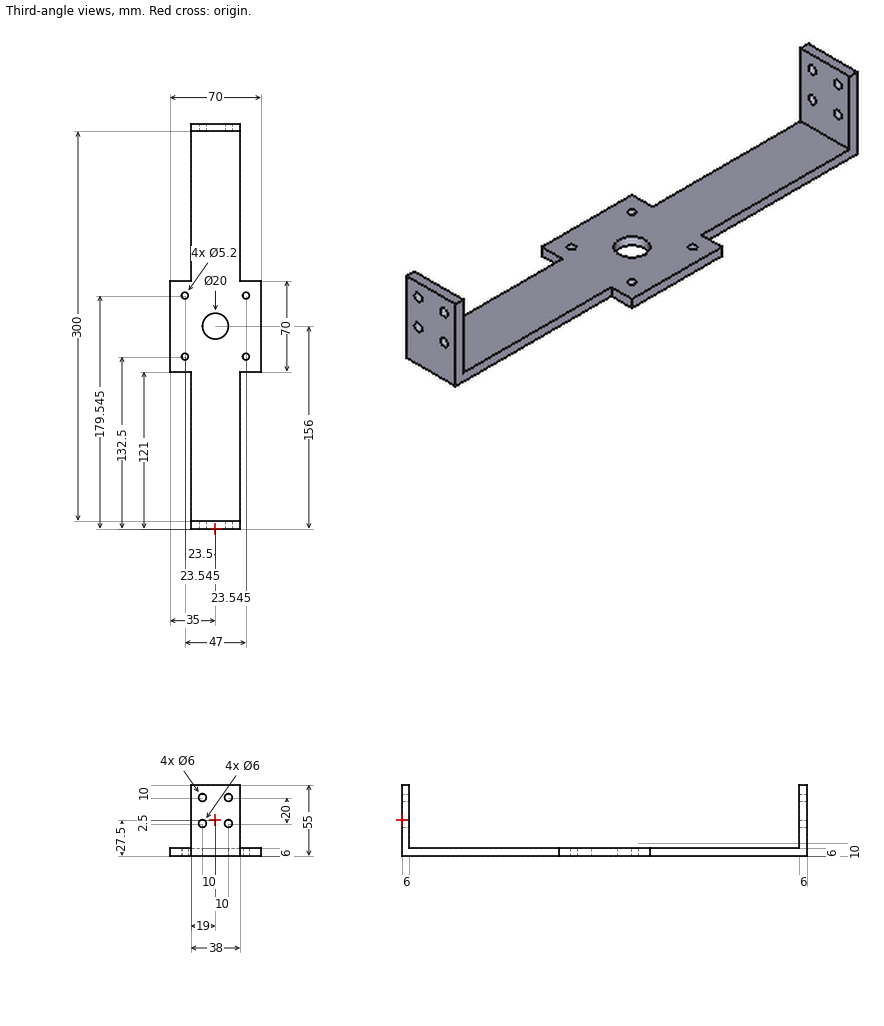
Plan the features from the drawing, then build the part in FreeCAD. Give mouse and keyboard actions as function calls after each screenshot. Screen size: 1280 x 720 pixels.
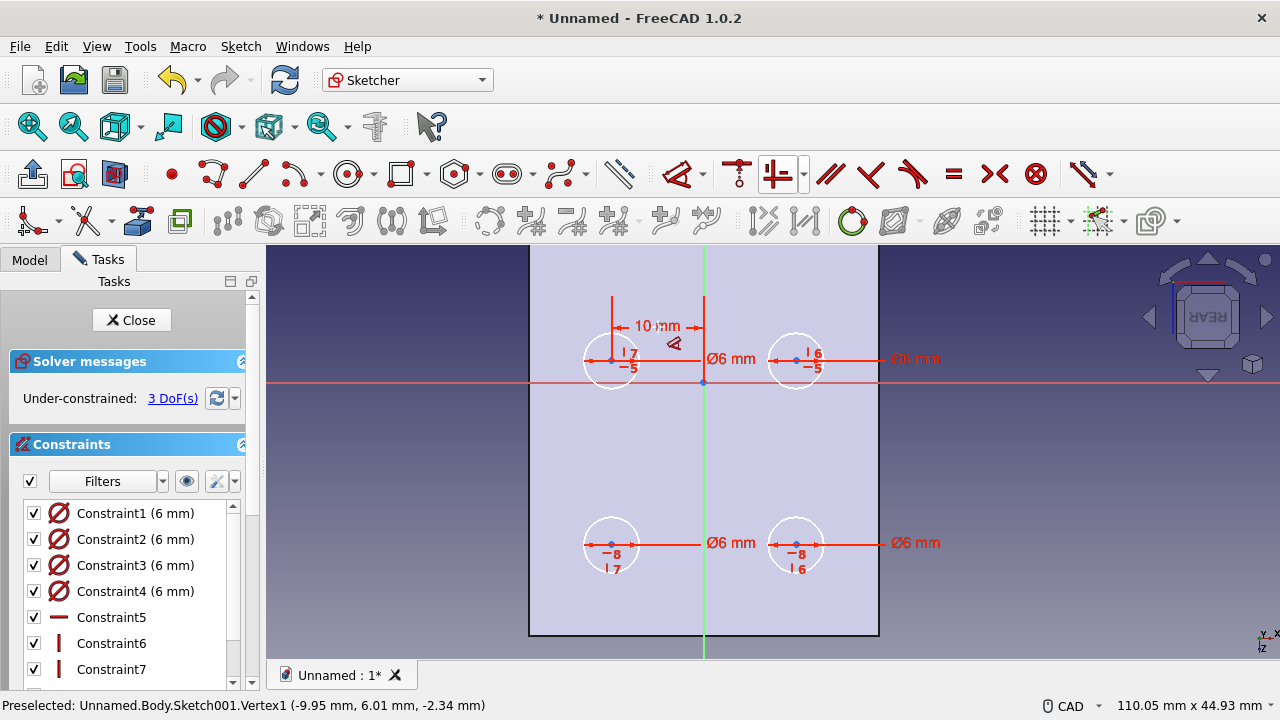
click(796, 361)
click(750, 327)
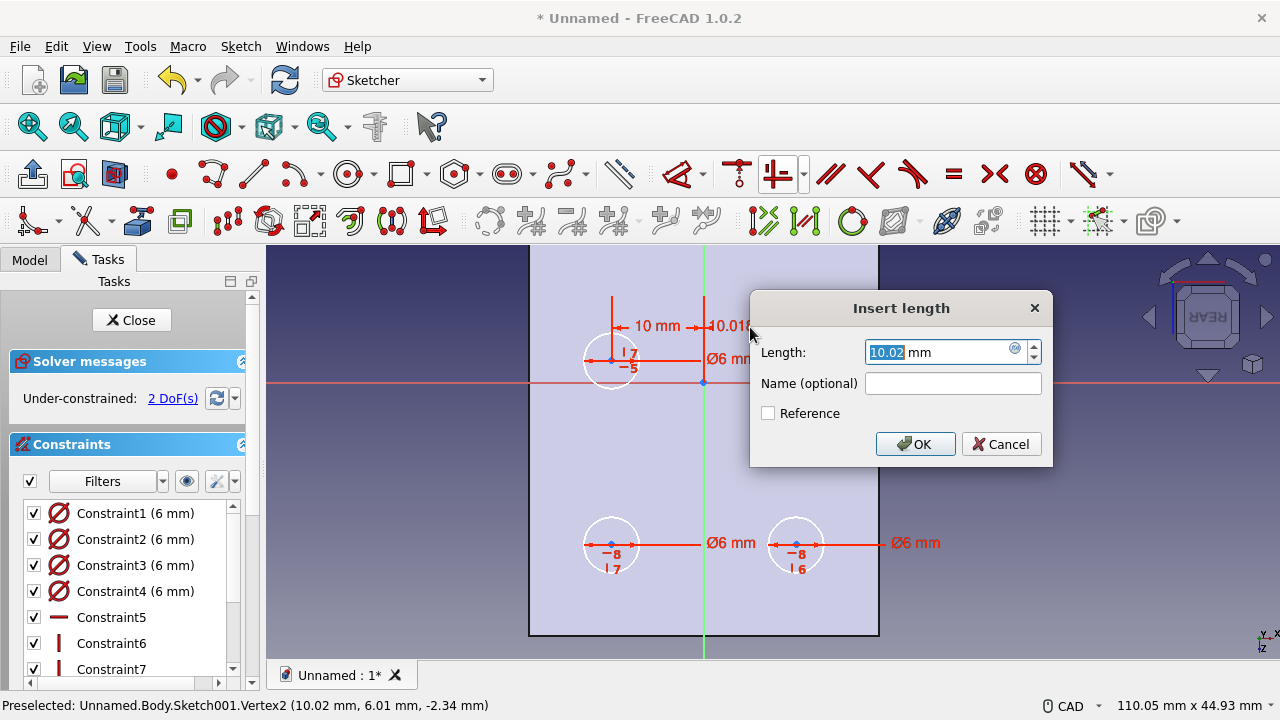
text(10)
key(Return)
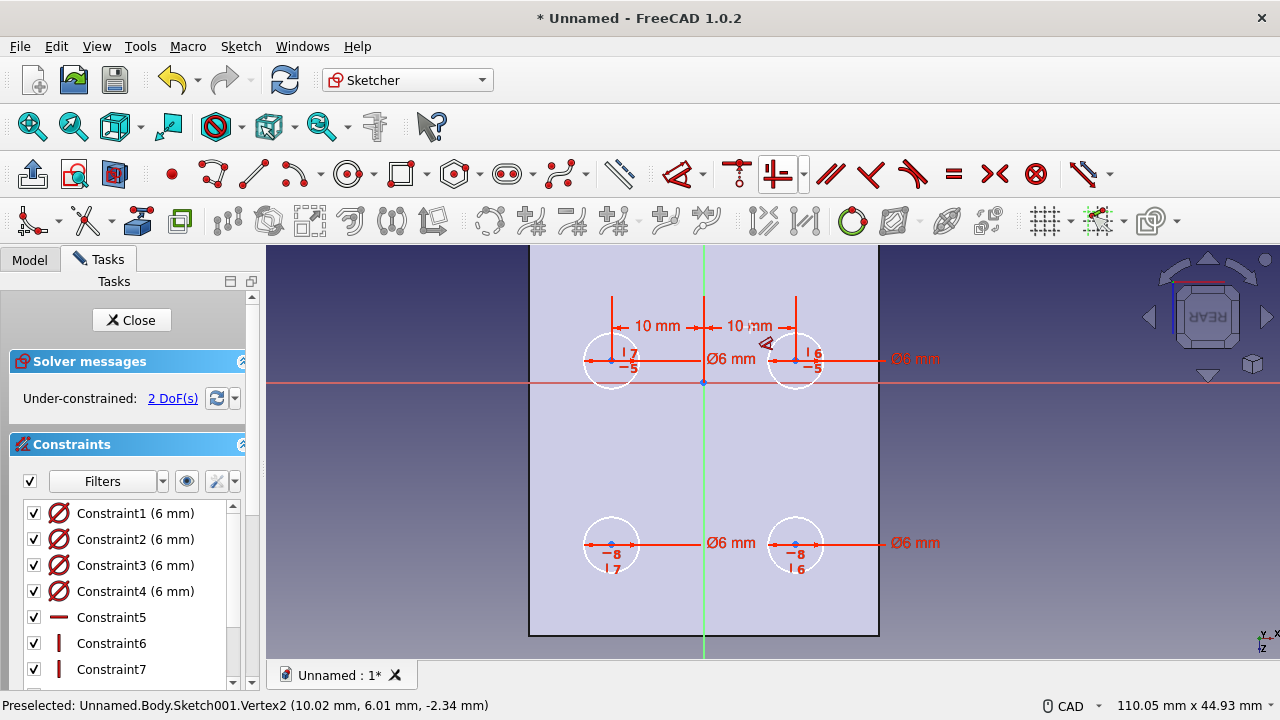
scroll(612, 361, up, 3)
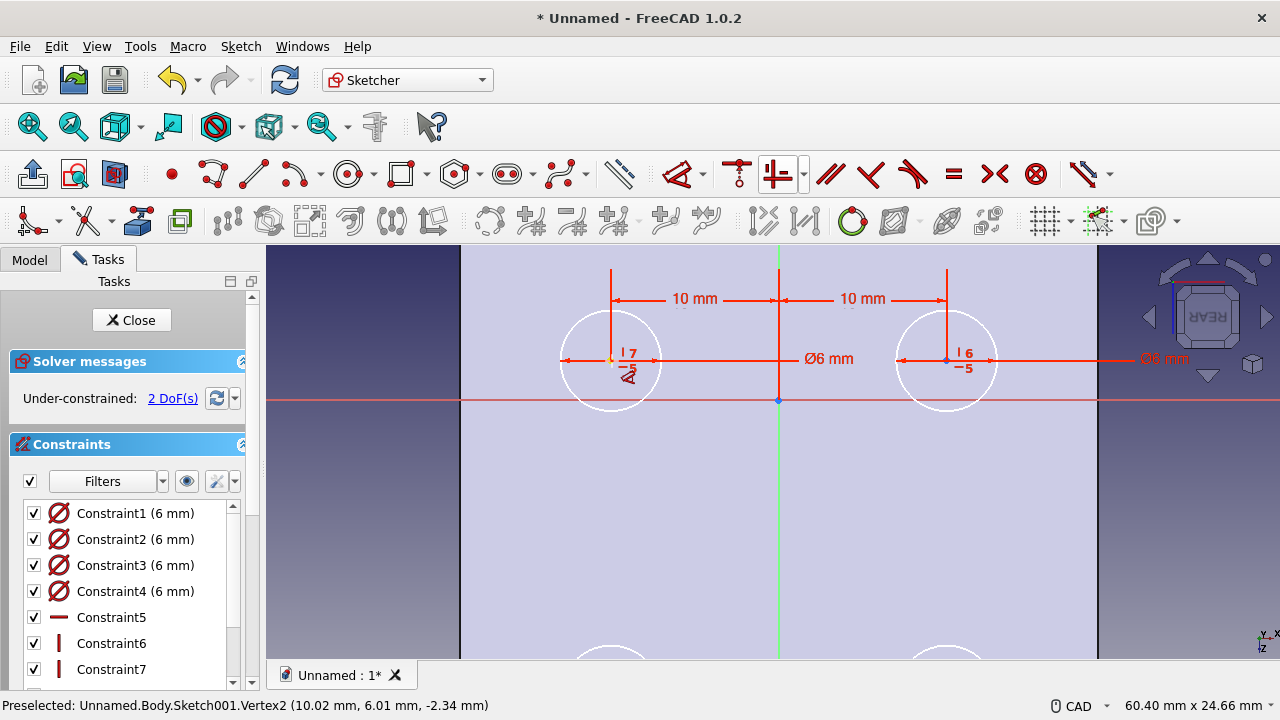
click(611, 361)
click(577, 371)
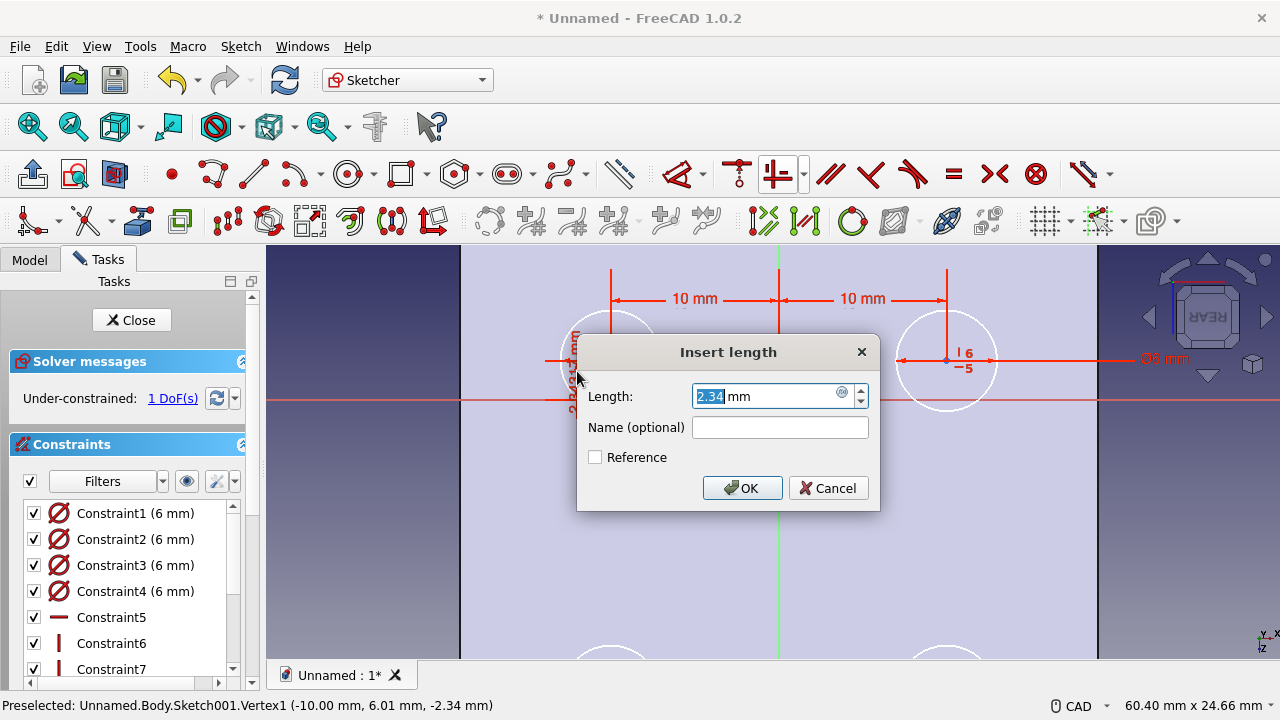
text(2.5)
key(Return)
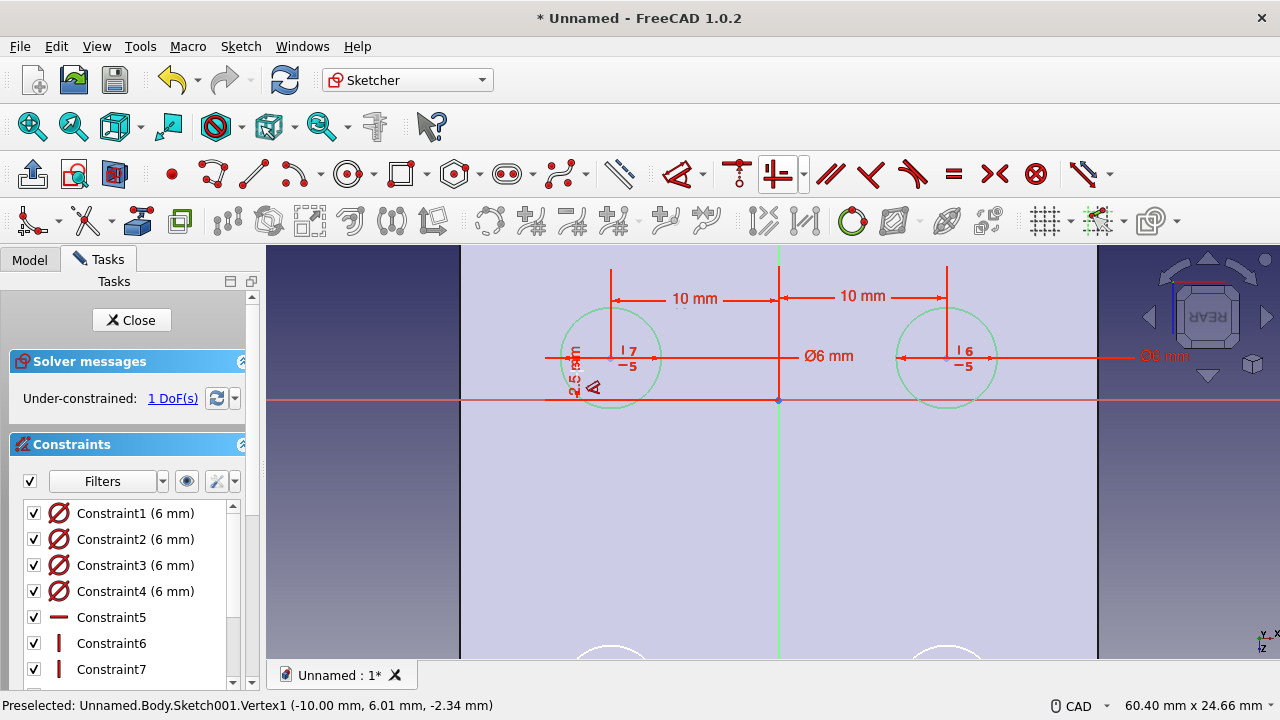
click(947, 358)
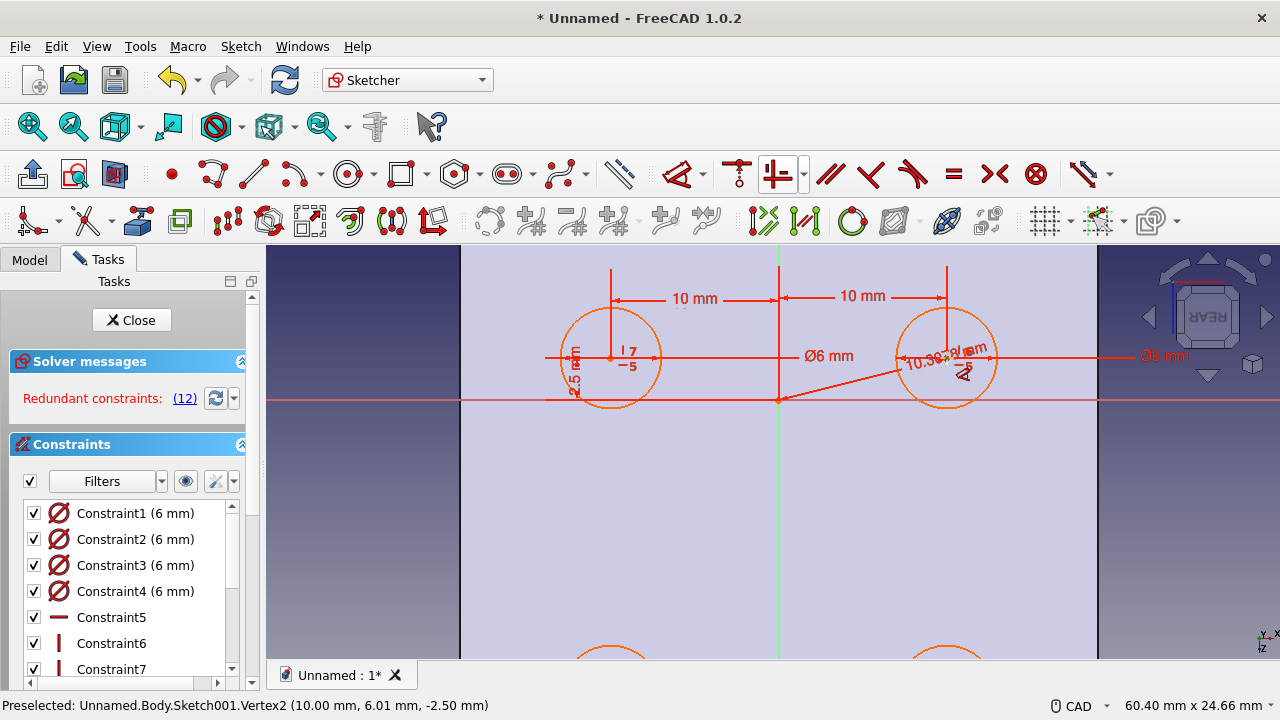
scroll(614, 362, down, 3)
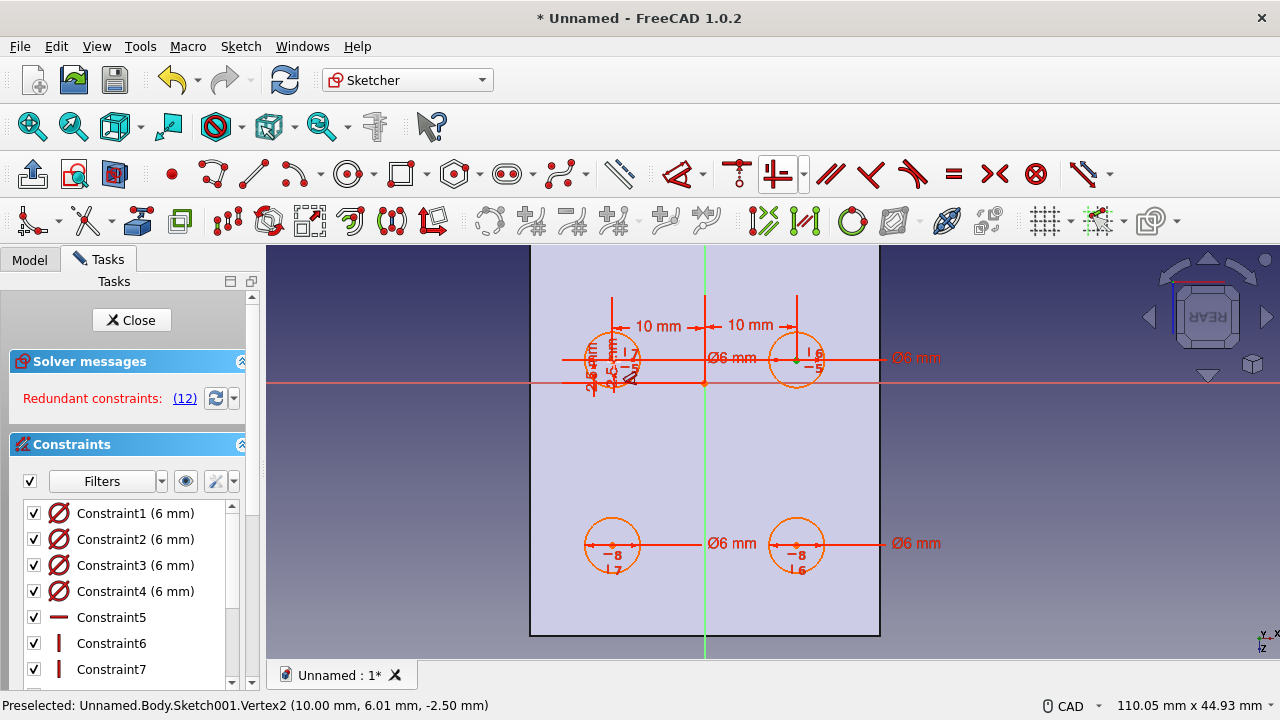
click(797, 545)
click(831, 453)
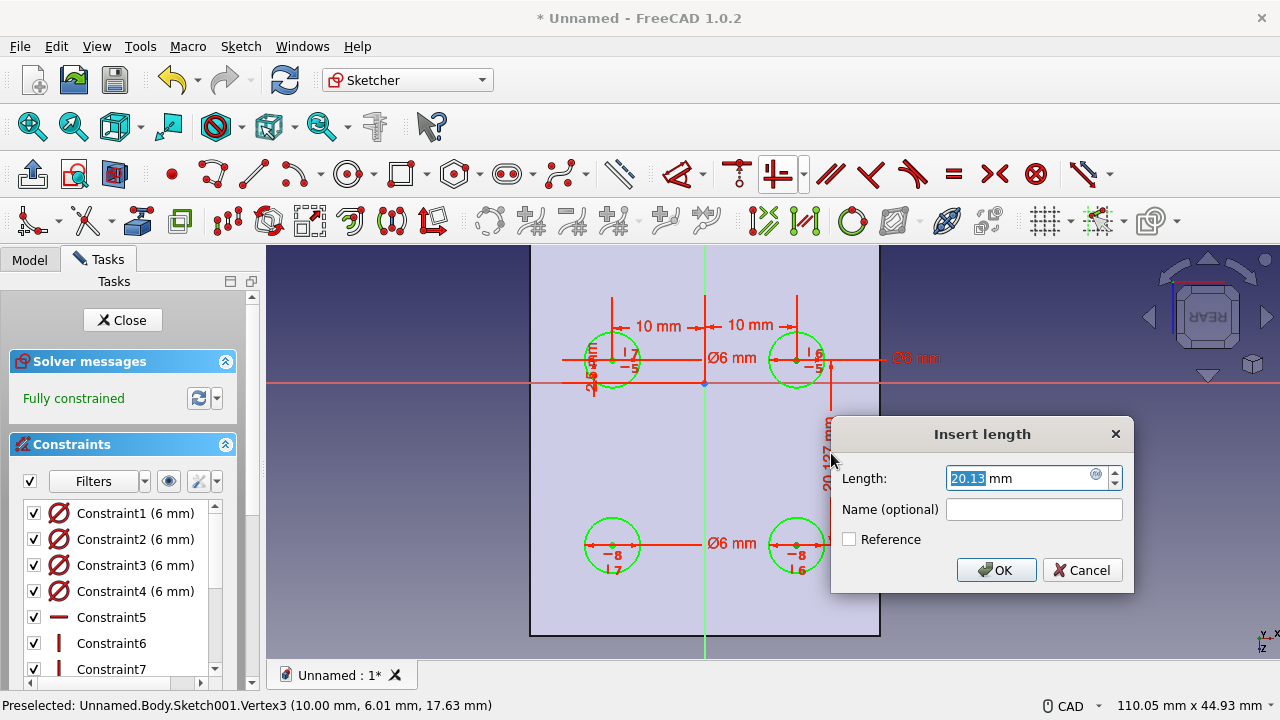
text(20)
key(Return)
key(Escape)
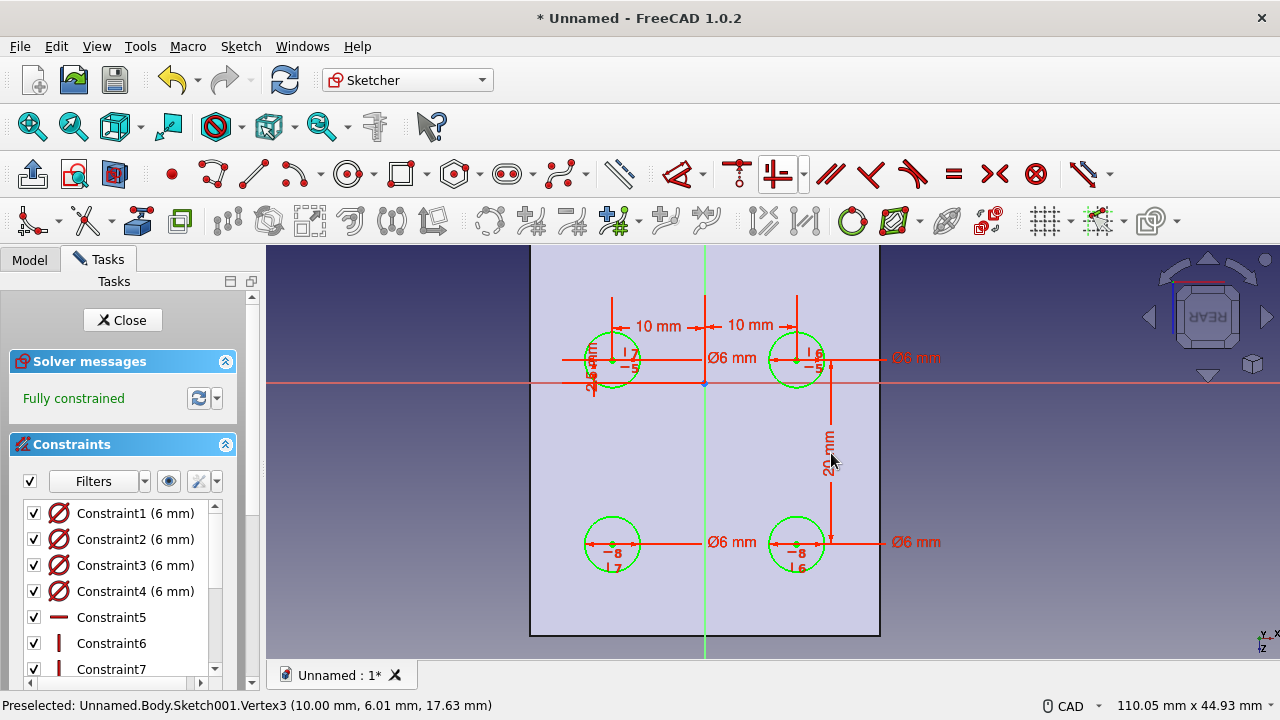
click(123, 320)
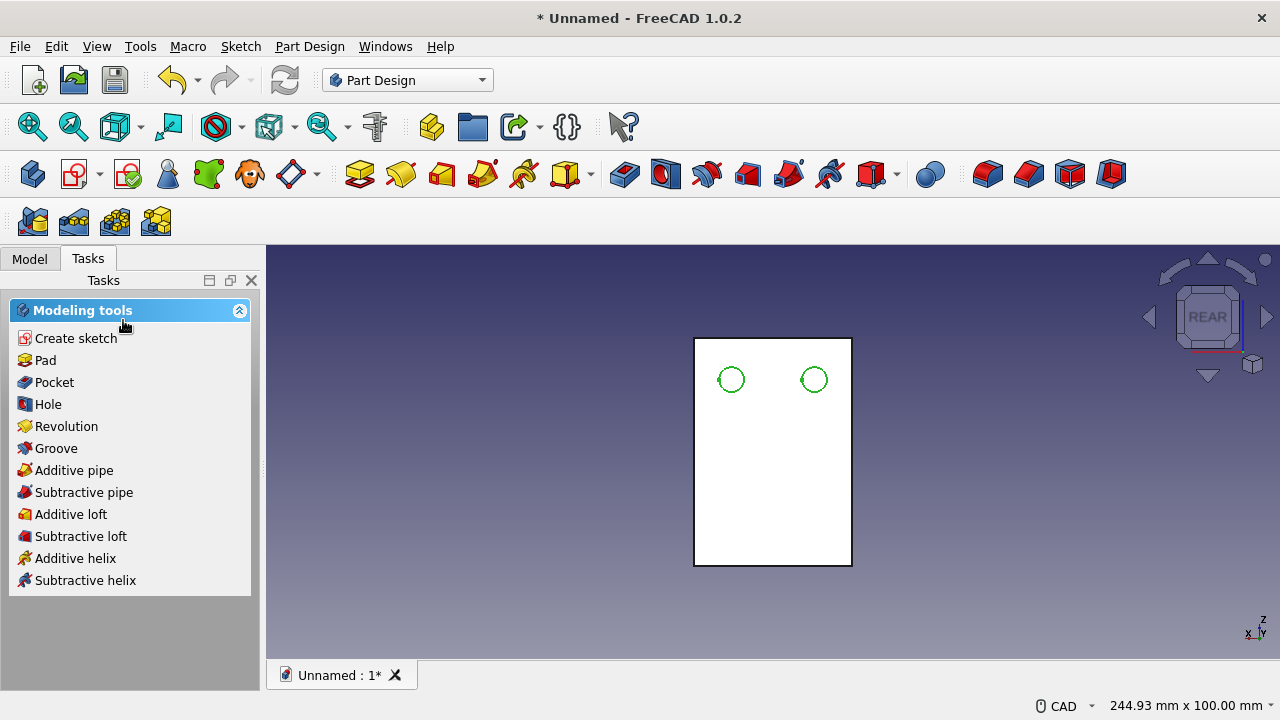
click(625, 174)